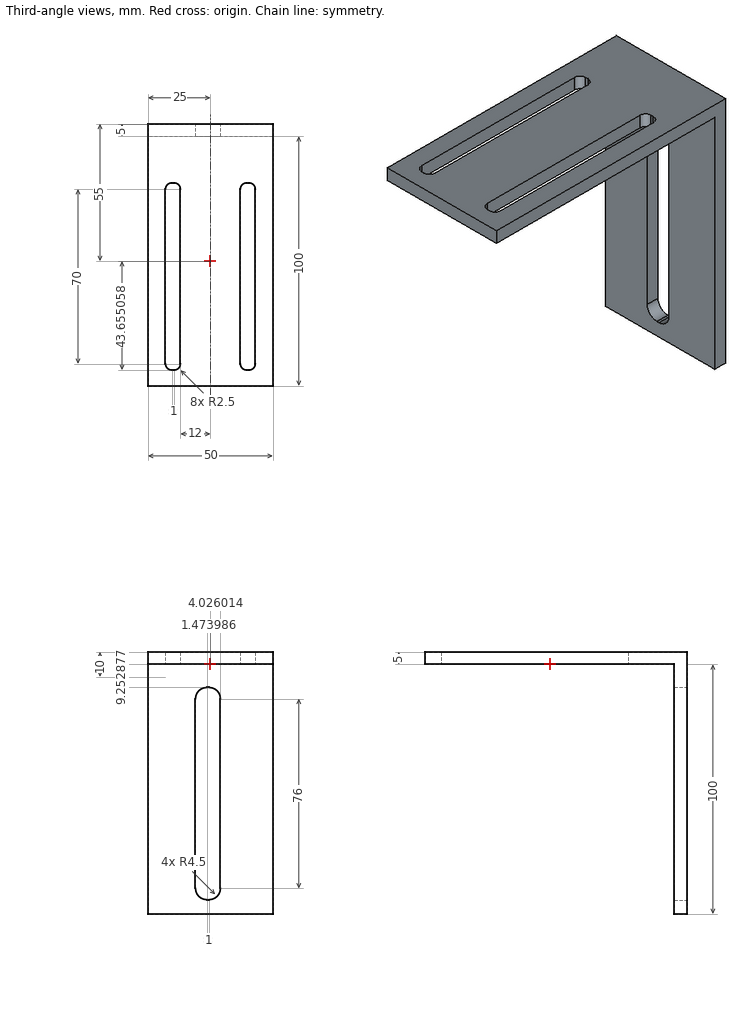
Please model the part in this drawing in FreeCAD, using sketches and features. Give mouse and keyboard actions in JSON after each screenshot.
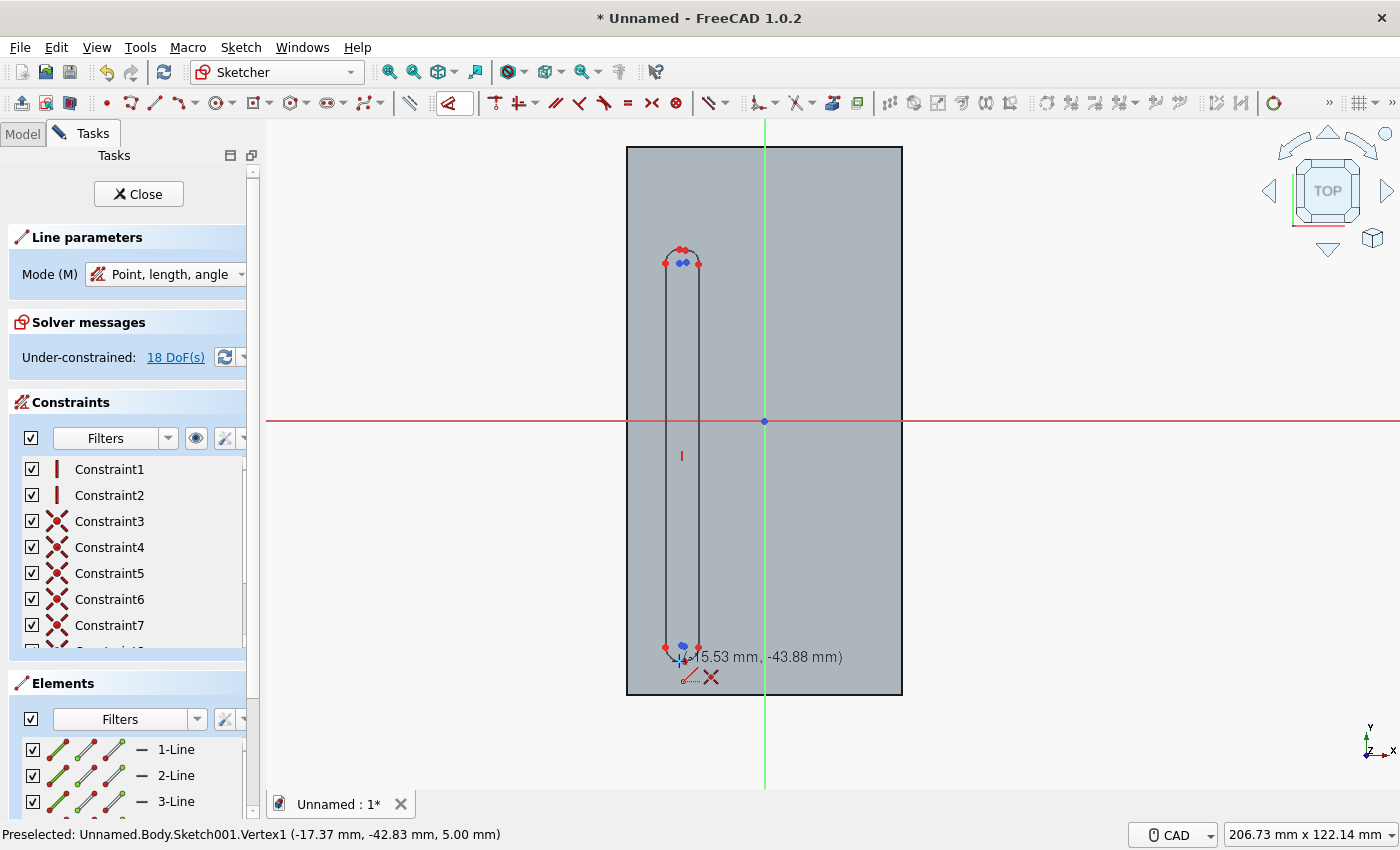
{"action": "left_click", "coordinate": [844, 661]}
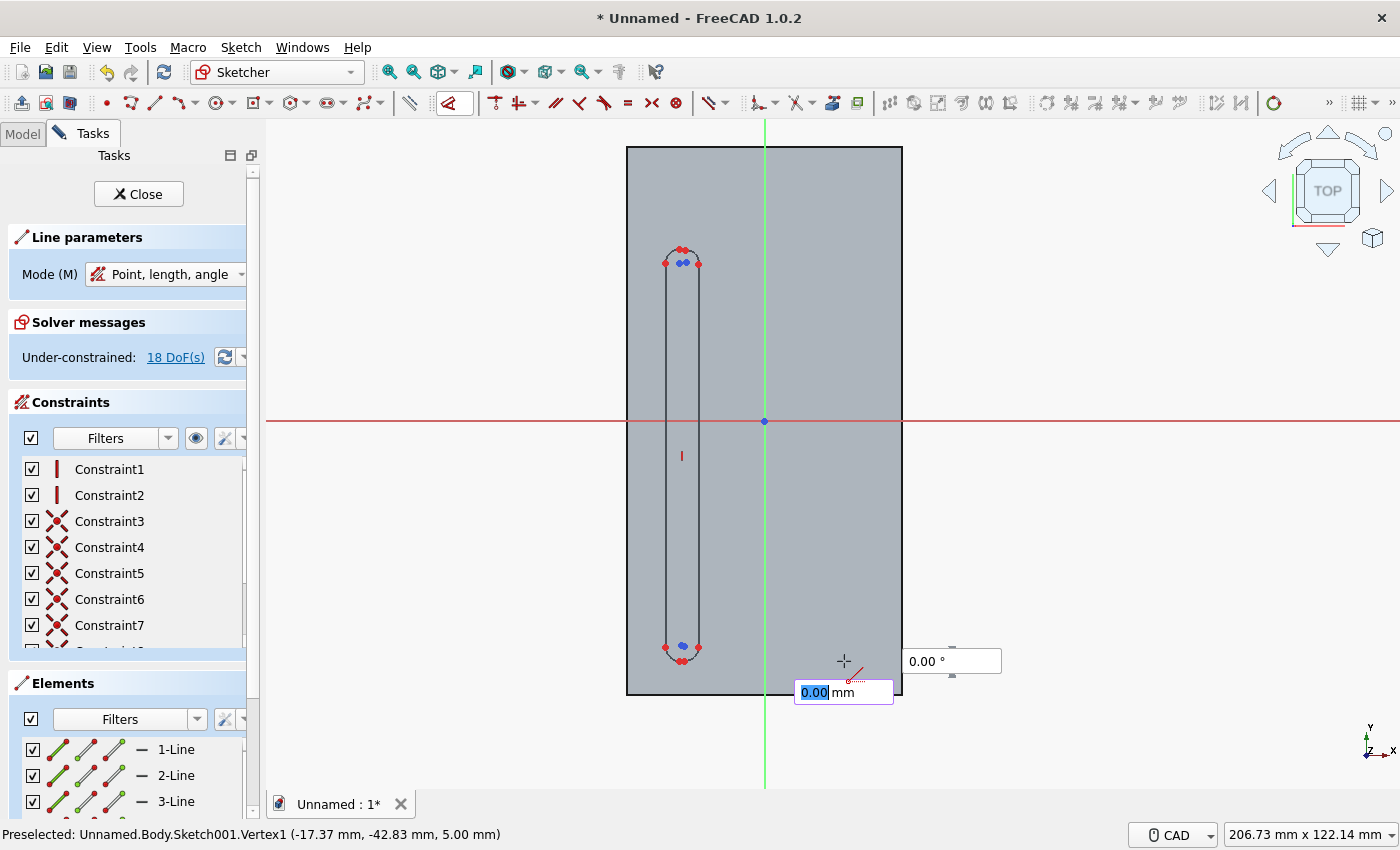
{"action": "scroll", "coordinate": [850, 661], "scroll_direction": "up", "scroll_amount": 6}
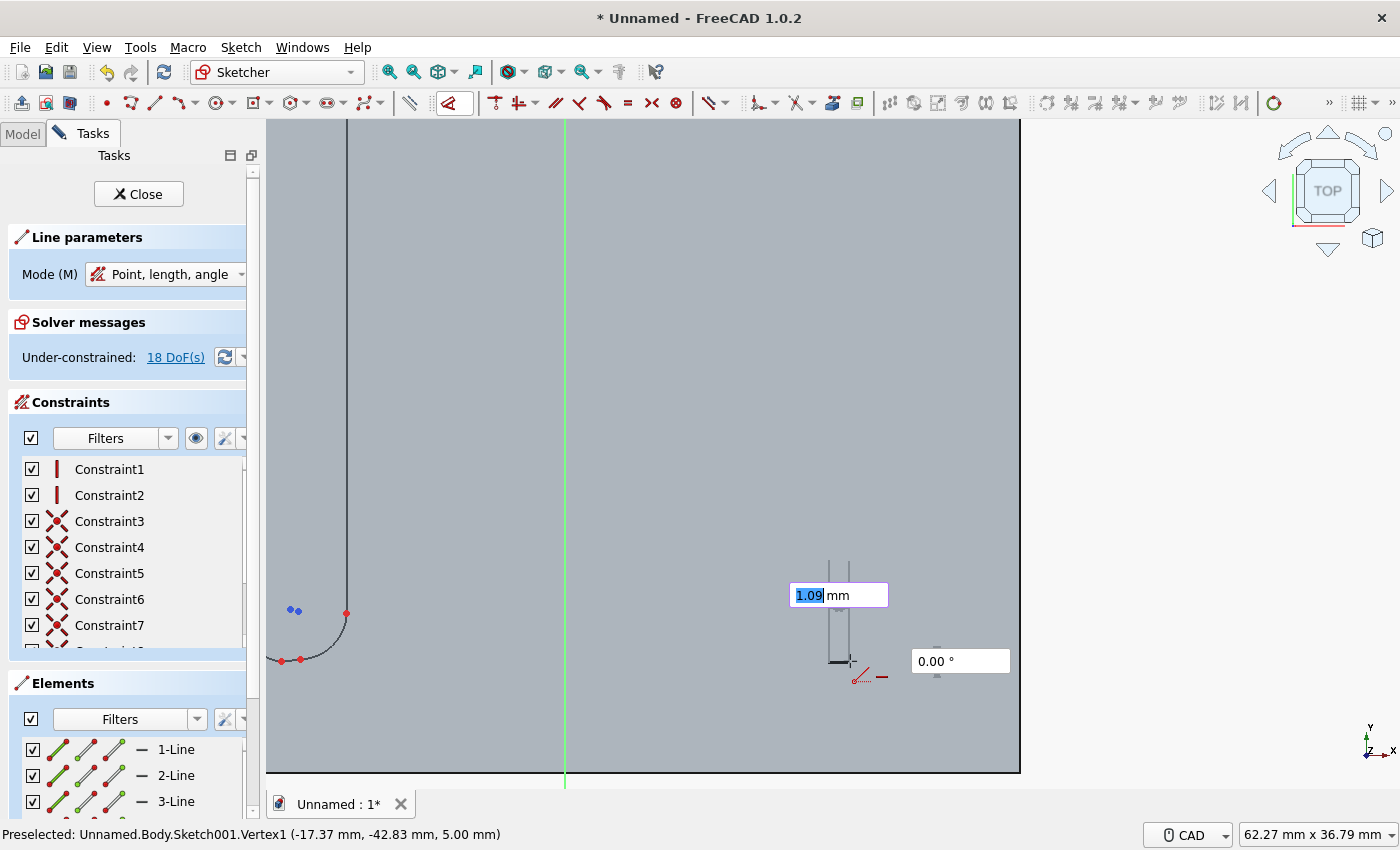
{"action": "left_click", "coordinate": [847, 659]}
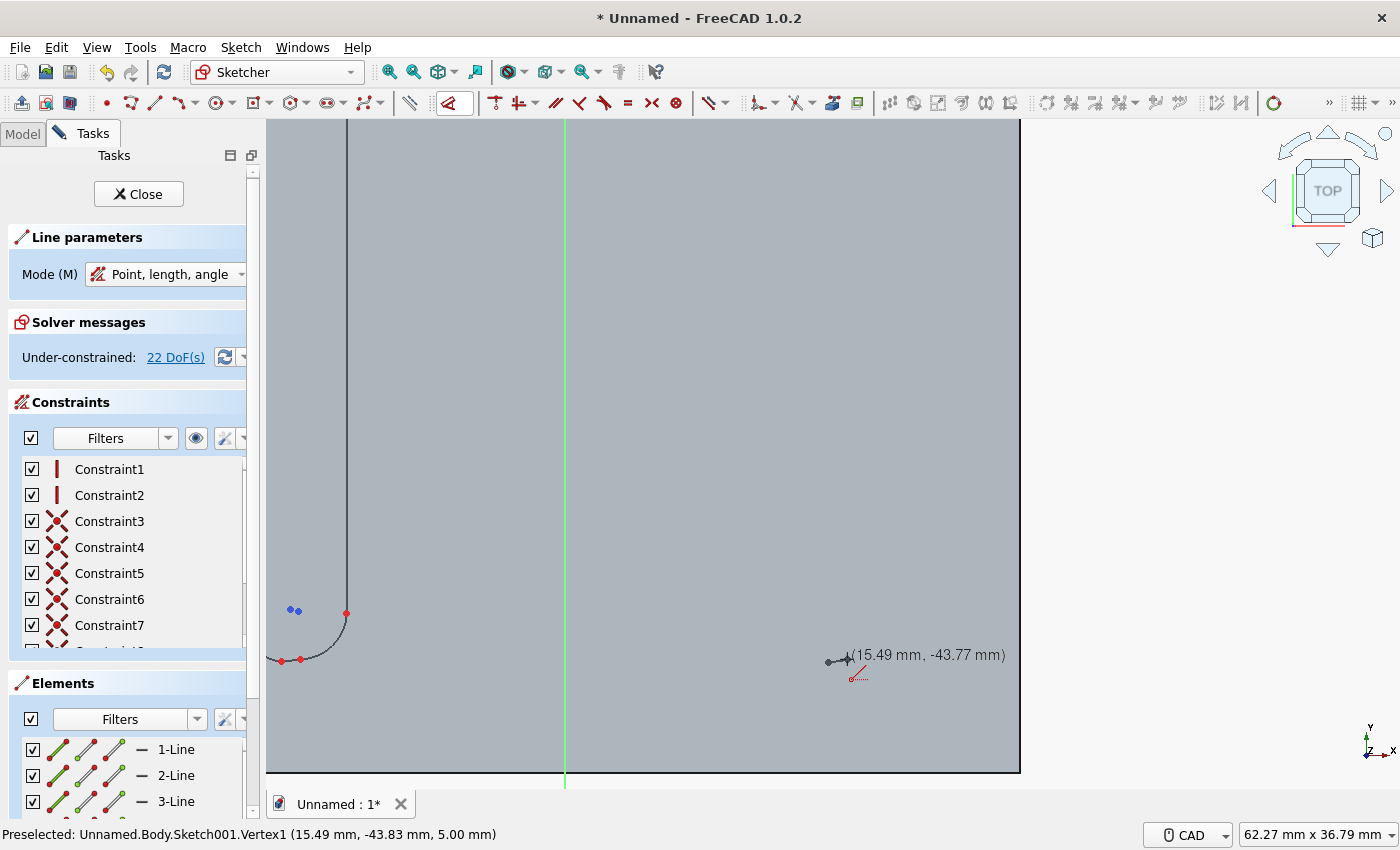
{"action": "left_click", "coordinate": [893, 612]}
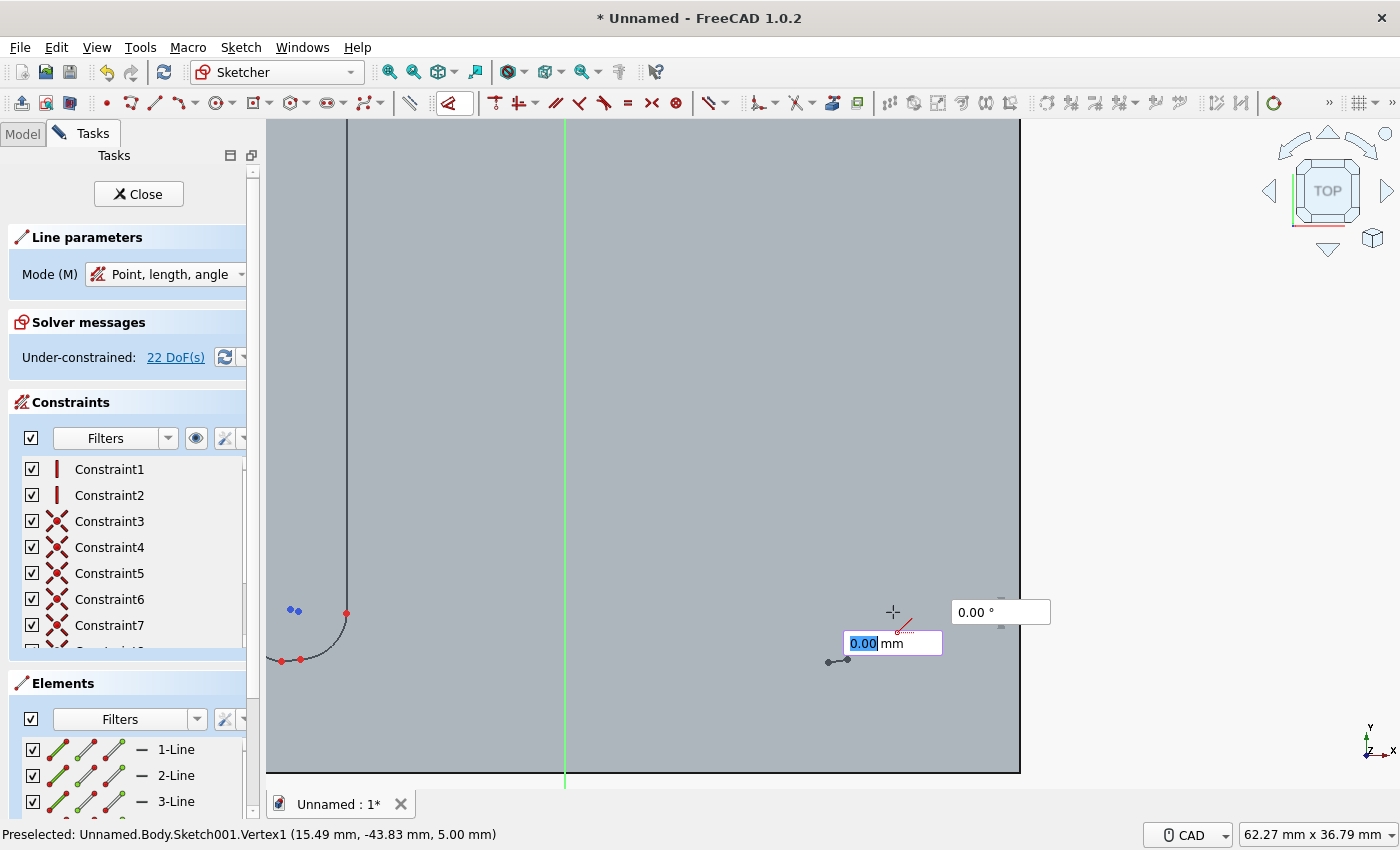
{"action": "scroll", "coordinate": [851, 660], "scroll_direction": "down", "scroll_amount": 6}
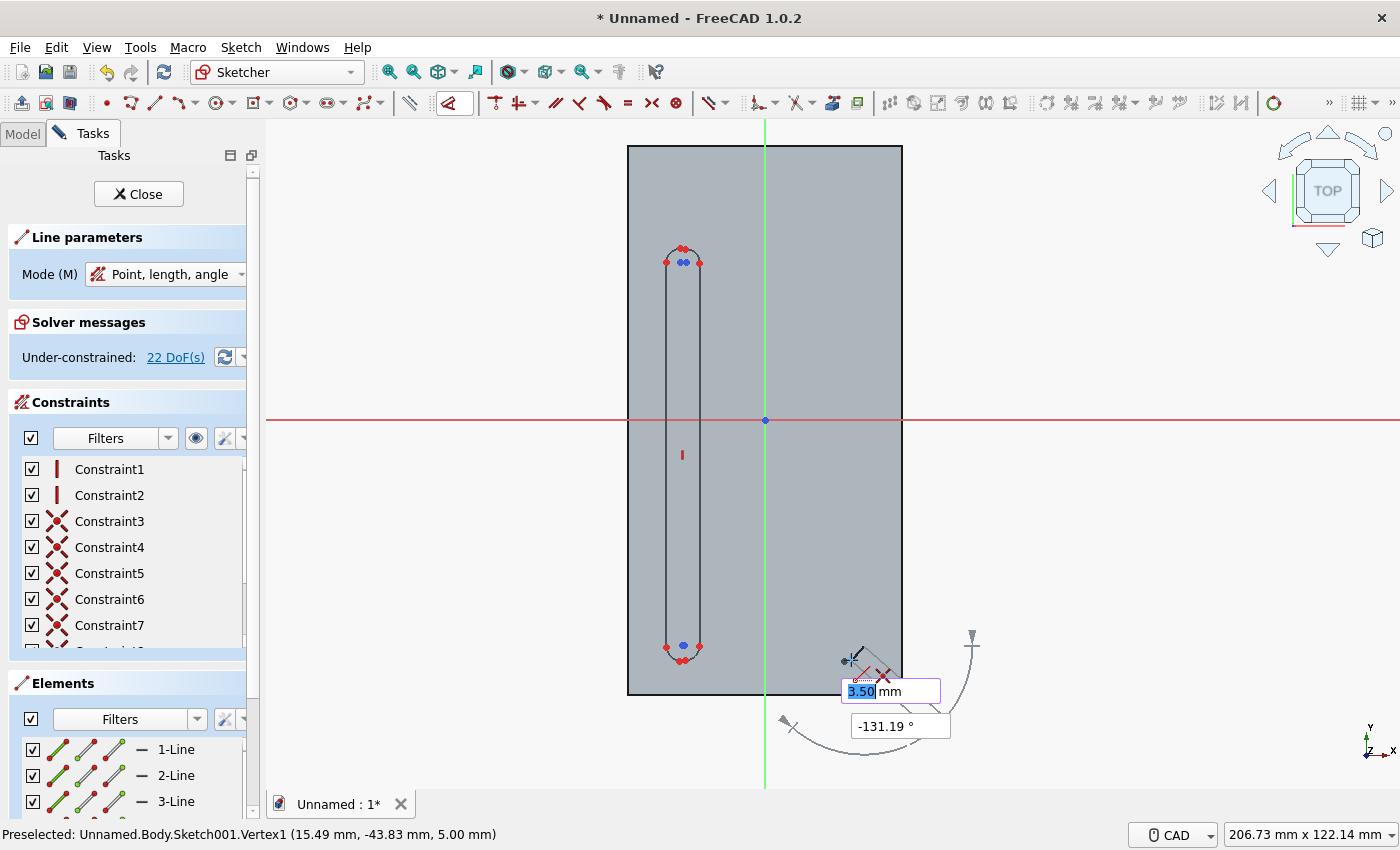
{"action": "left_click", "coordinate": [864, 262]}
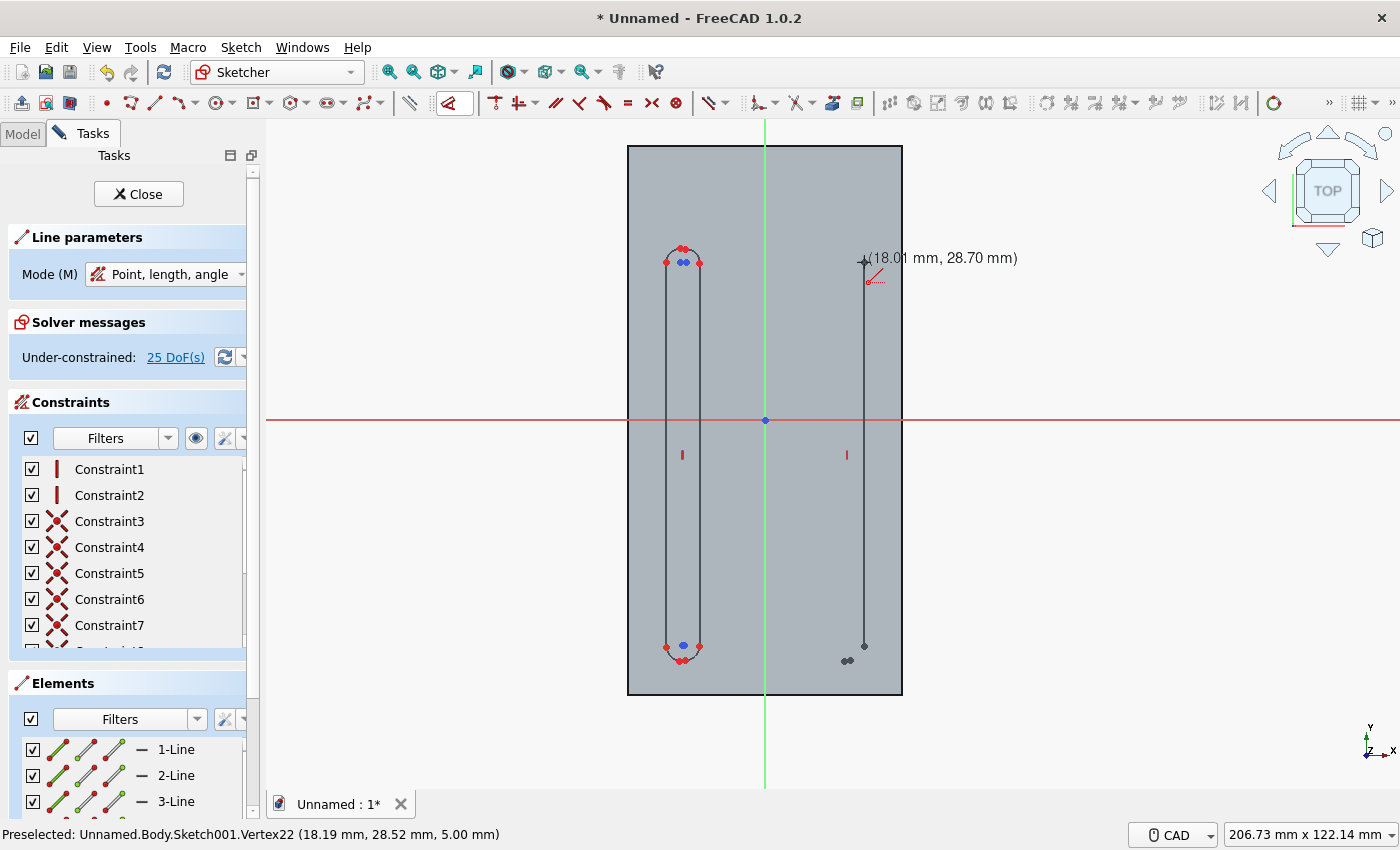
{"action": "left_click", "coordinate": [850, 249]}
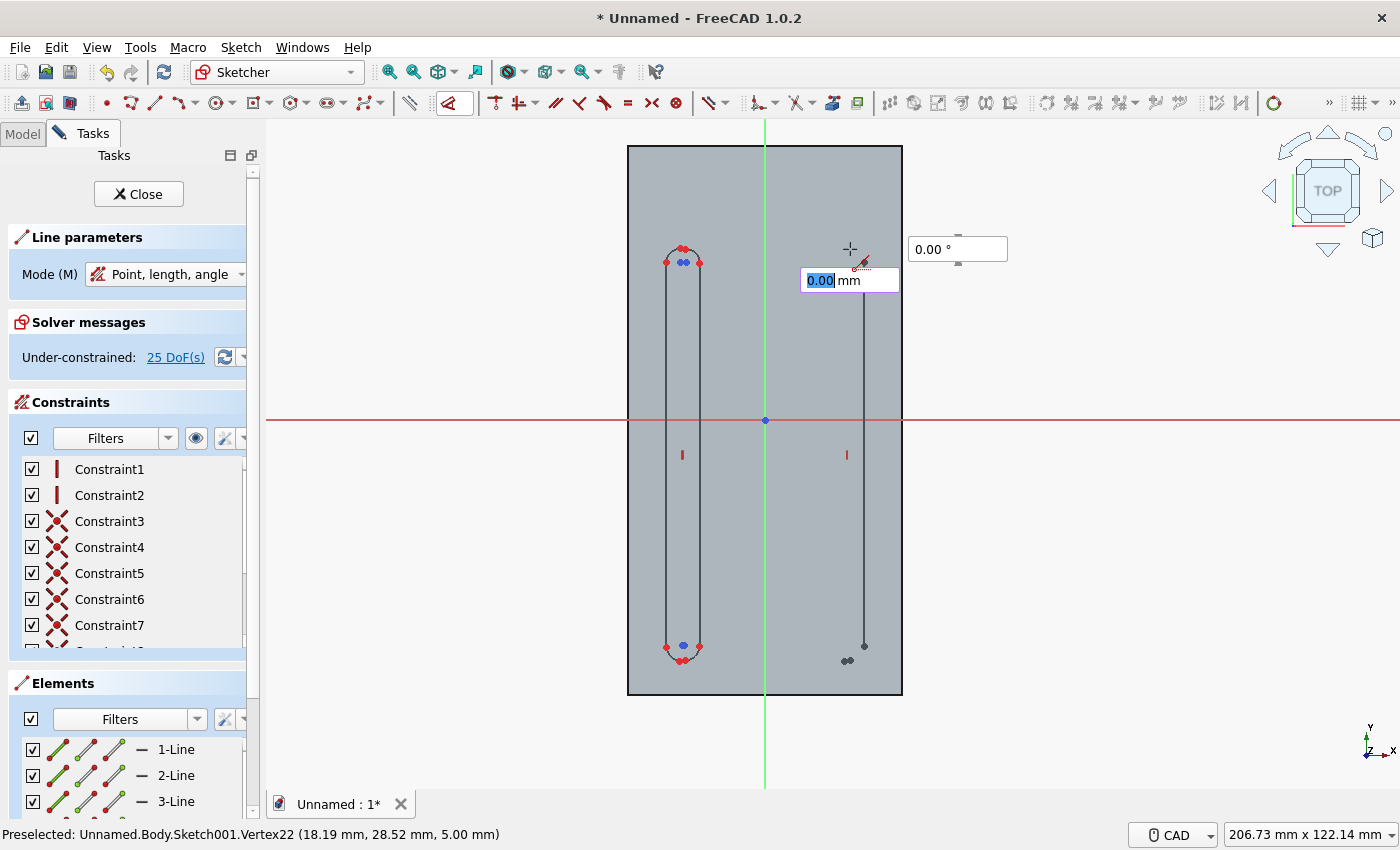
{"action": "scroll", "coordinate": [845, 249], "scroll_direction": "up", "scroll_amount": 6}